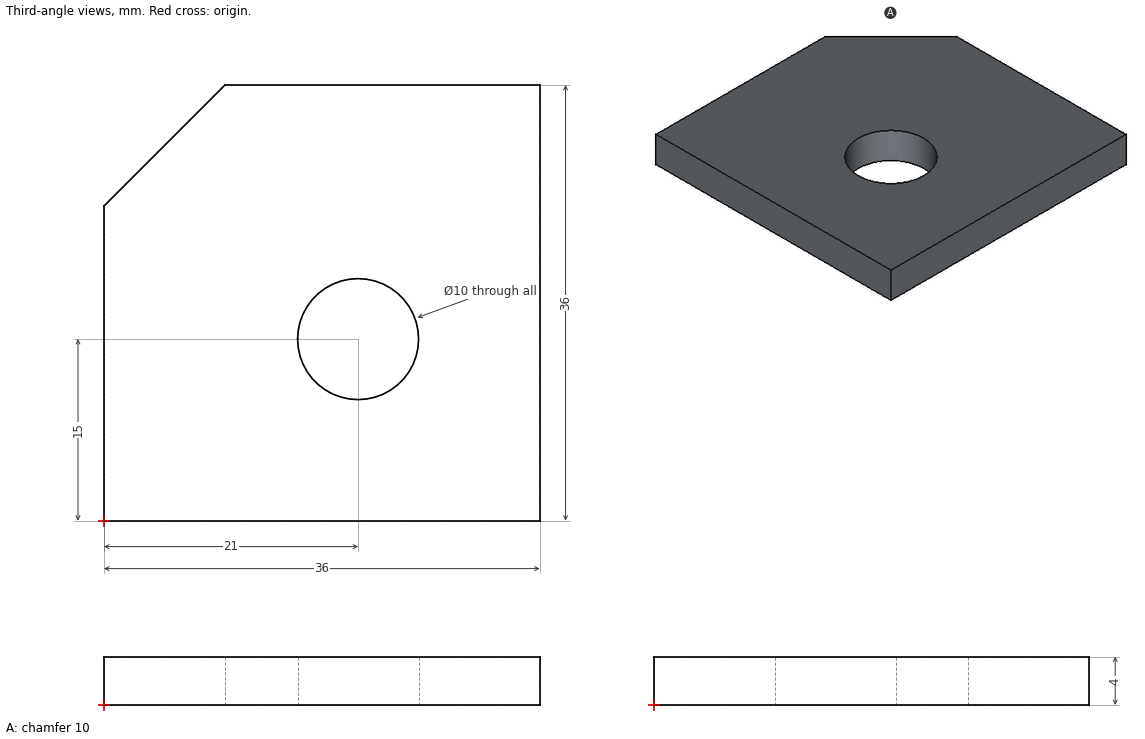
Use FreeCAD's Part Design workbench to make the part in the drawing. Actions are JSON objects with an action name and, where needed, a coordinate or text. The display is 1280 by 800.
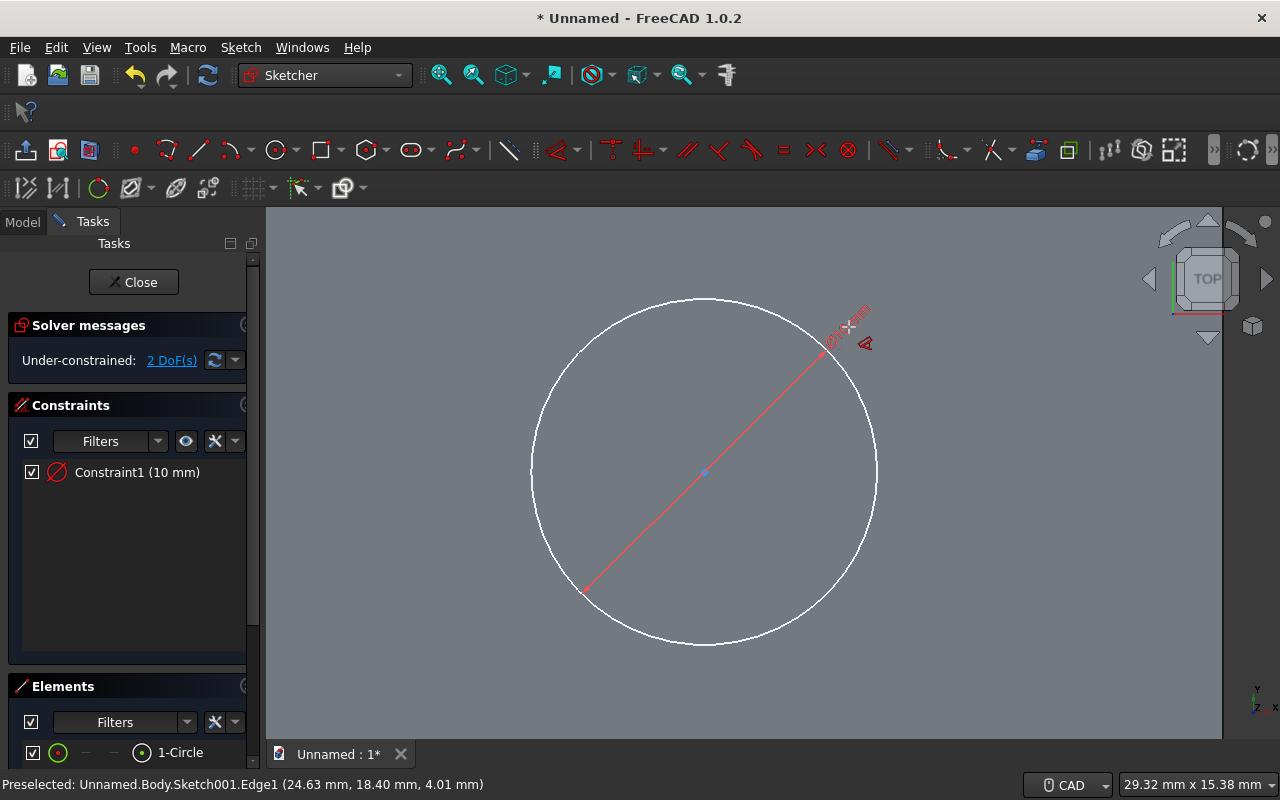
{"action": "left_click", "coordinate": [704, 472]}
{"action": "left_click", "coordinate": [499, 438]}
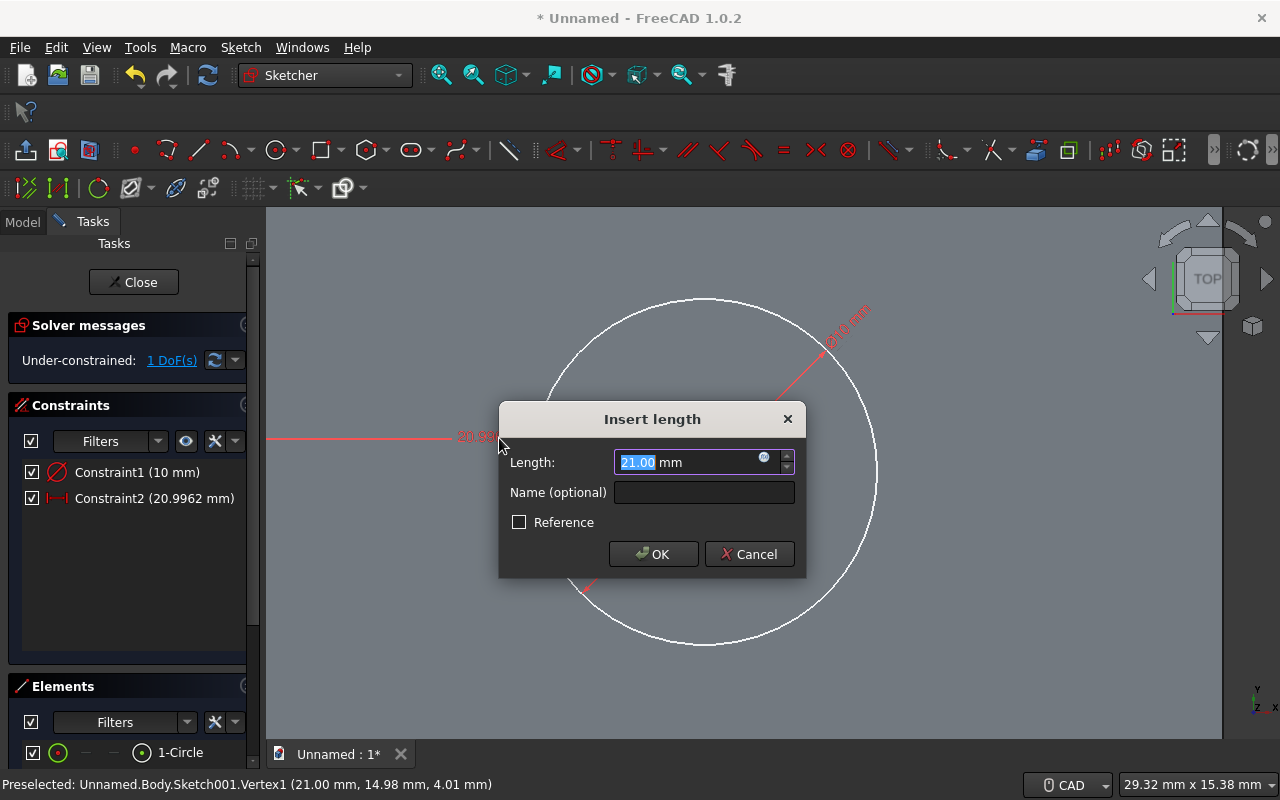
{"action": "type", "text": "21"}
{"action": "key", "text": "Return"}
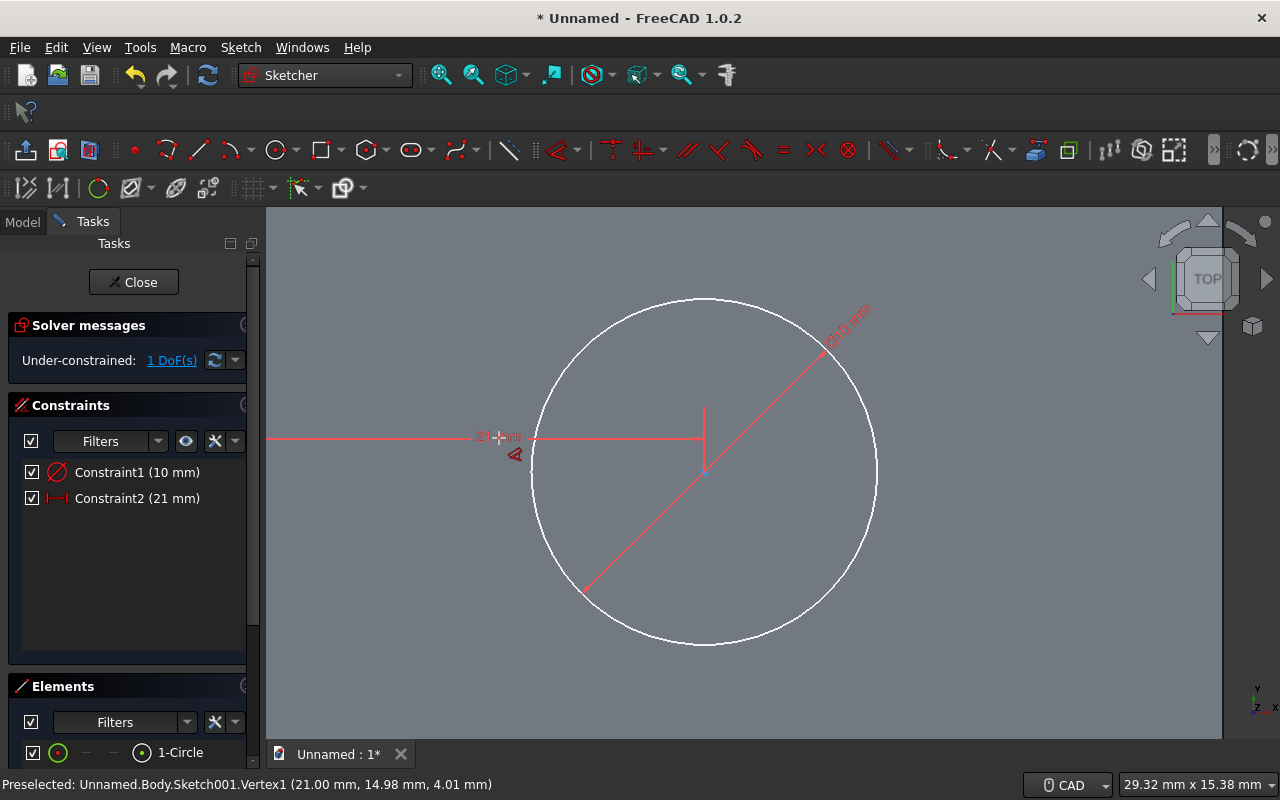
{"action": "left_click", "coordinate": [704, 472]}
{"action": "left_click", "coordinate": [738, 592]}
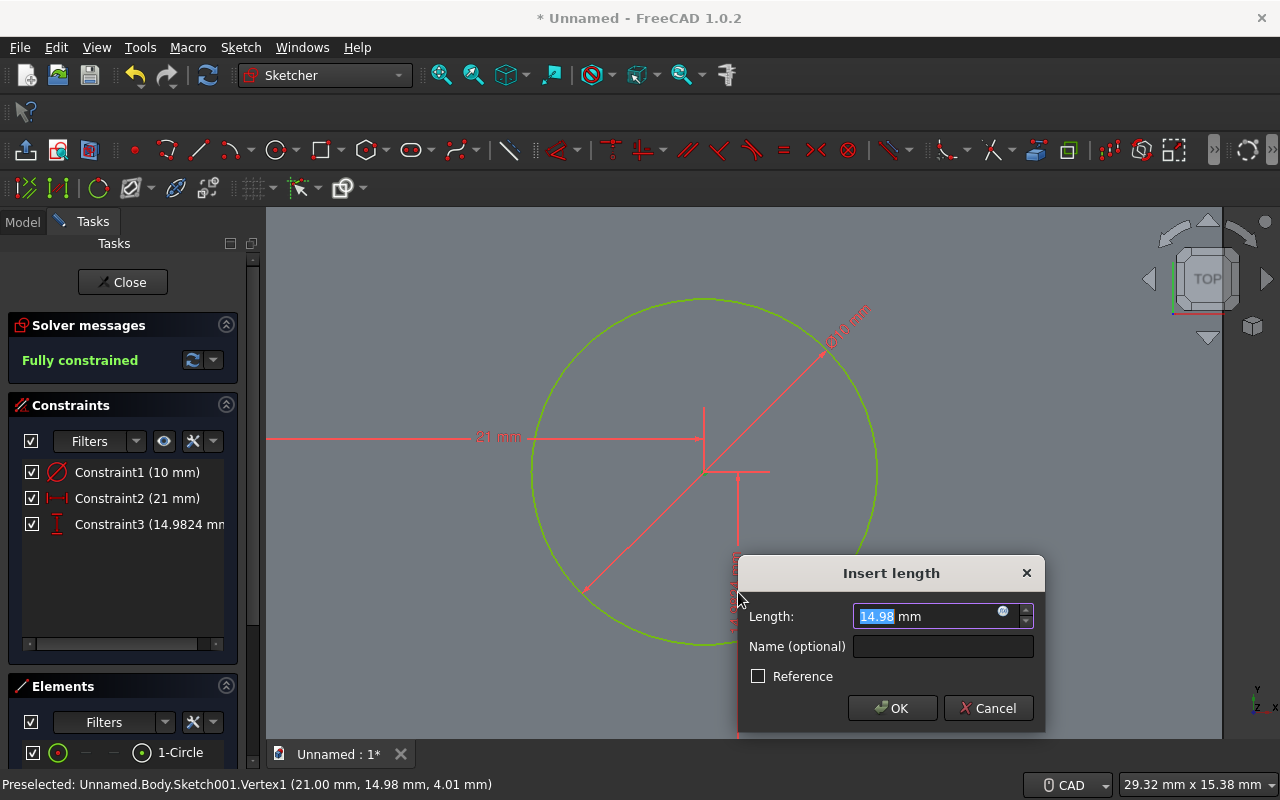
{"action": "type", "text": "15"}
{"action": "key", "text": "Return"}
{"action": "key", "text": "Escape"}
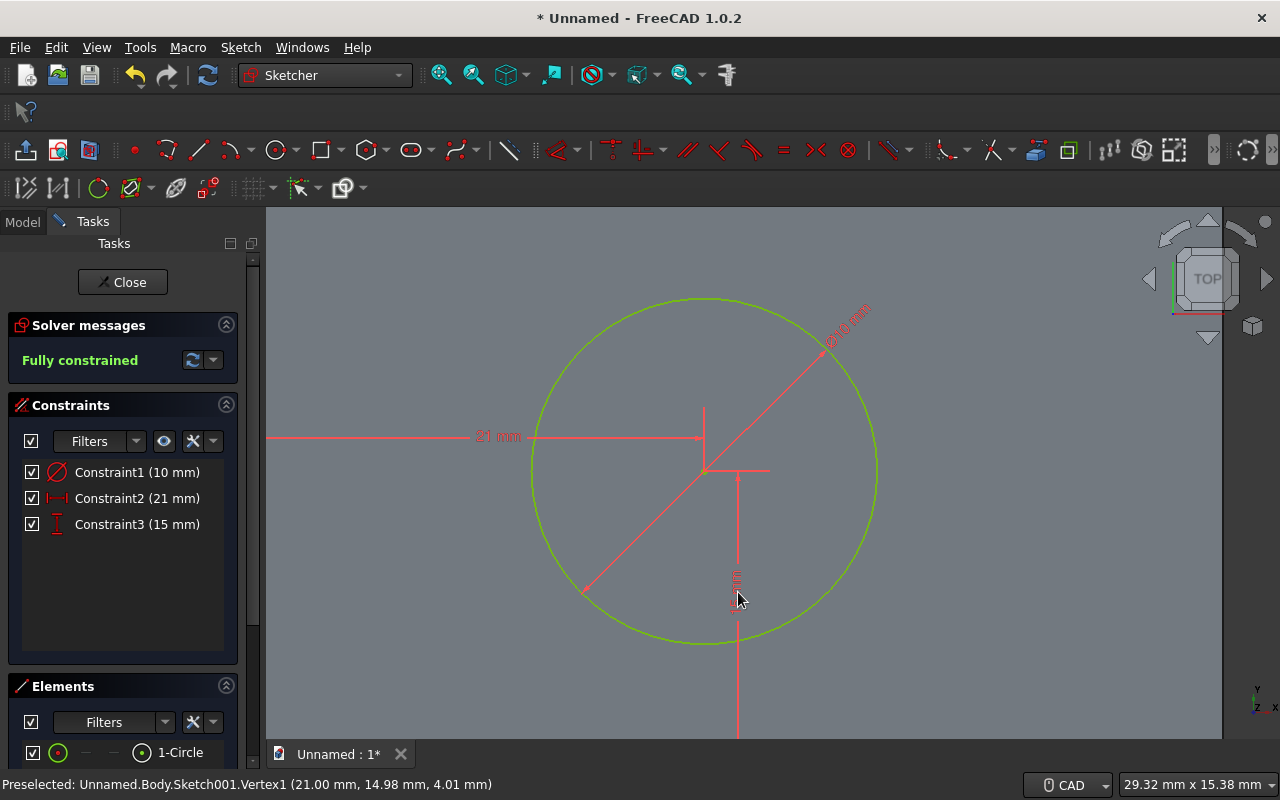
{"action": "left_click", "coordinate": [123, 282]}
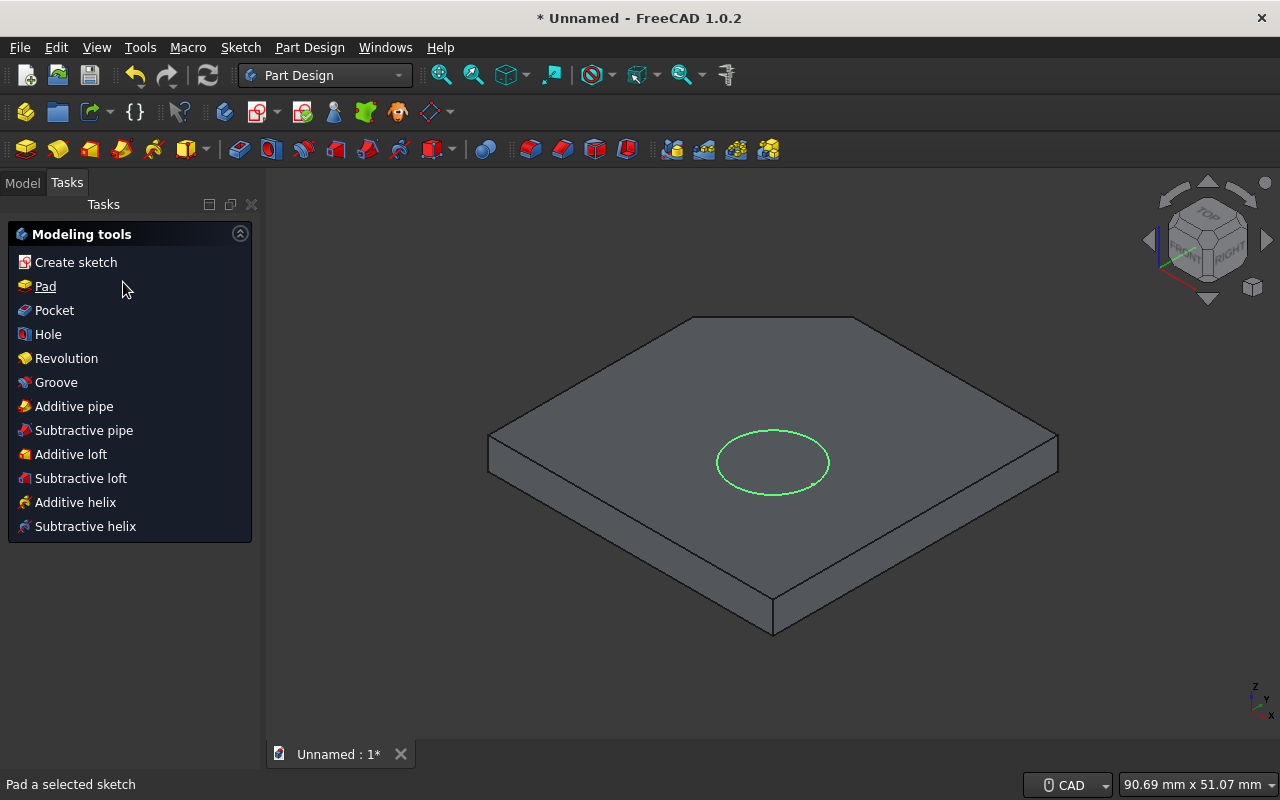
{"action": "left_click", "coordinate": [272, 150]}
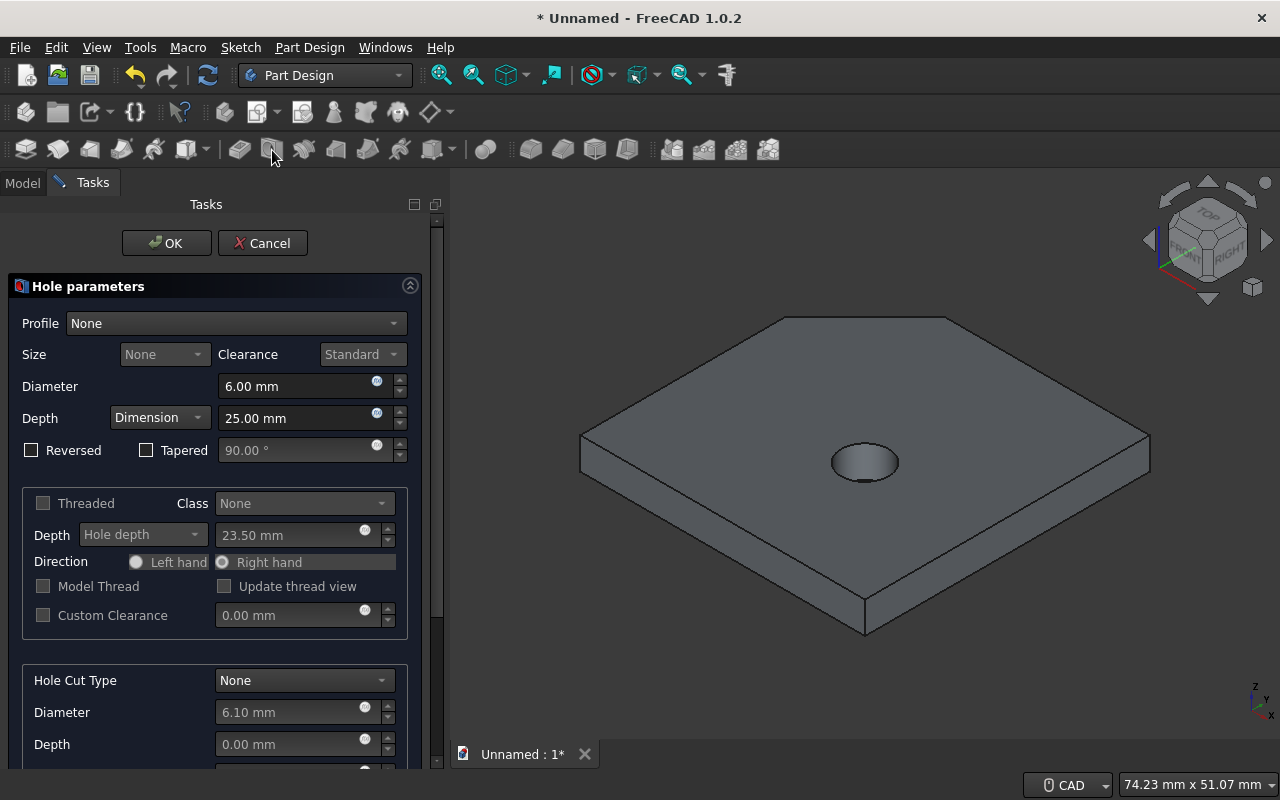
{"action": "triple_click", "coordinate": [305, 386]}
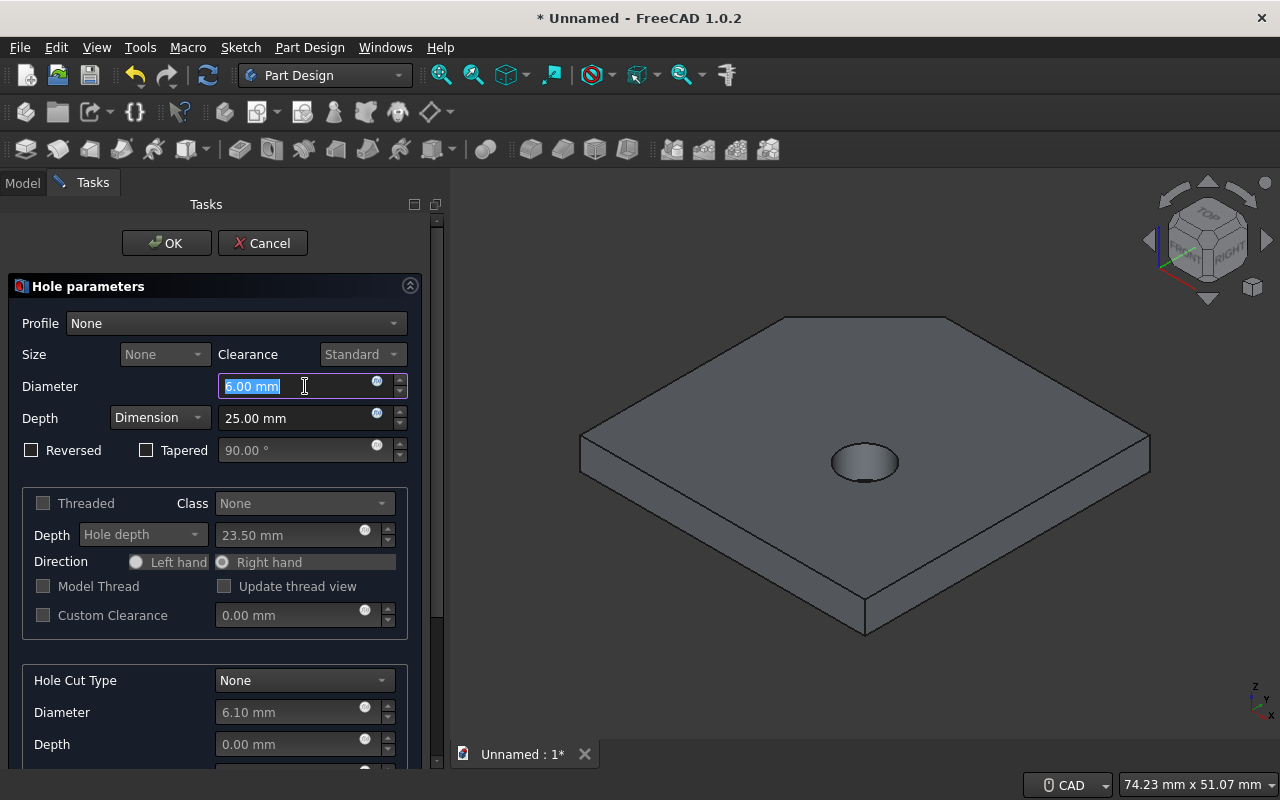
{"action": "type", "text": "10"}
{"action": "key", "text": "Tab"}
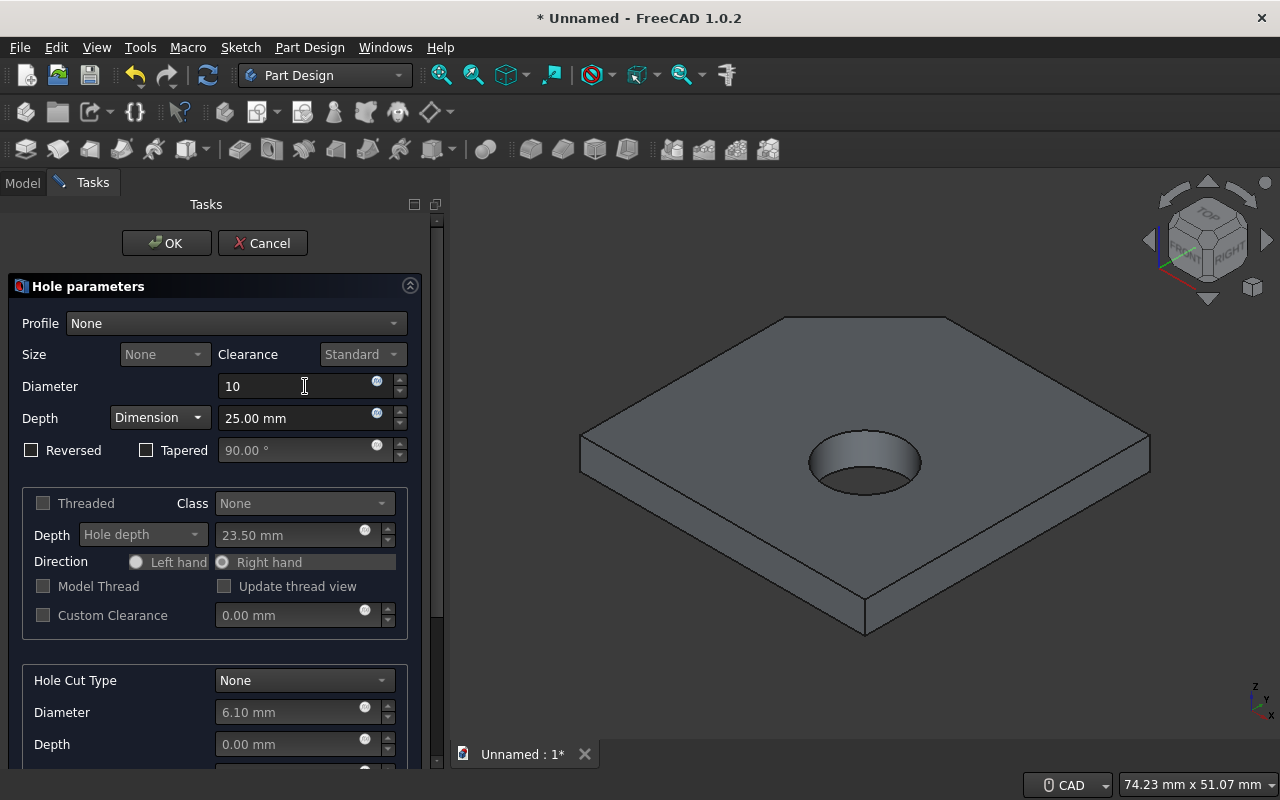
{"action": "left_click", "coordinate": [161, 418]}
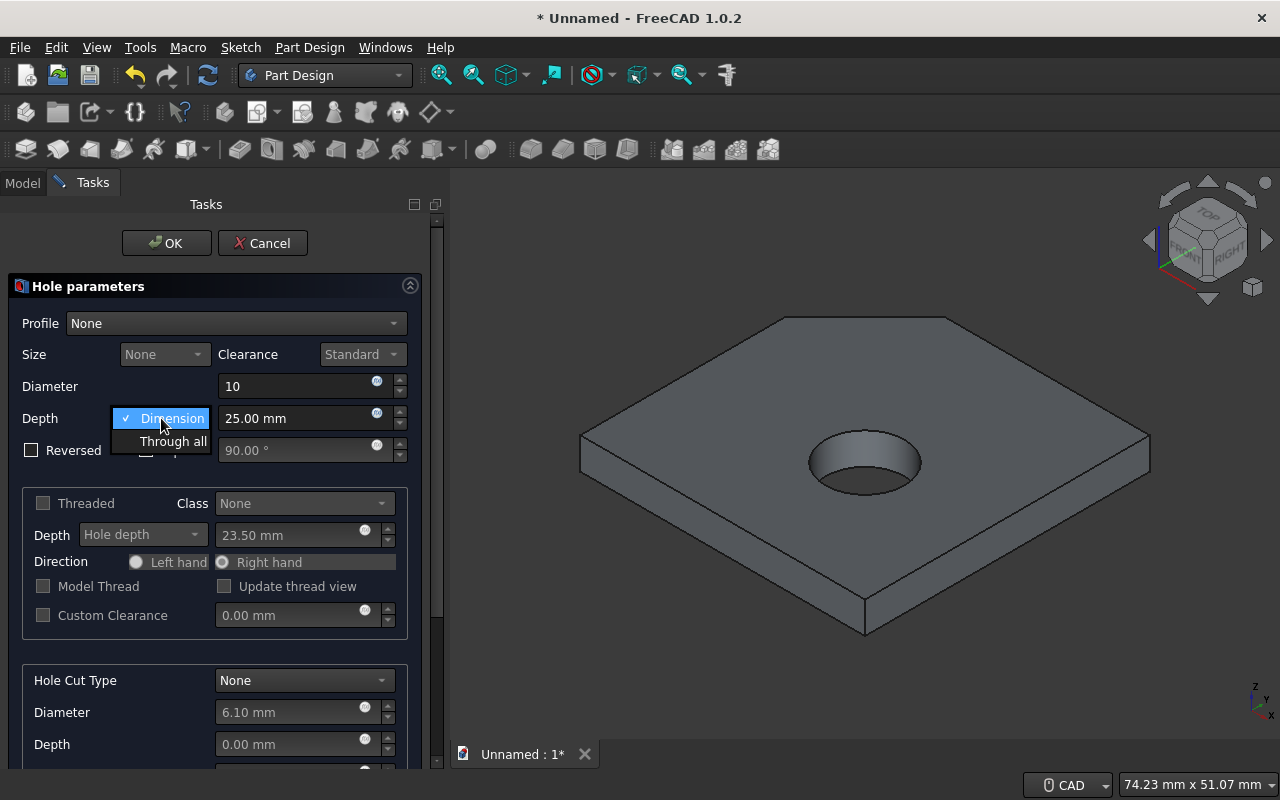
{"action": "left_click", "coordinate": [160, 442]}